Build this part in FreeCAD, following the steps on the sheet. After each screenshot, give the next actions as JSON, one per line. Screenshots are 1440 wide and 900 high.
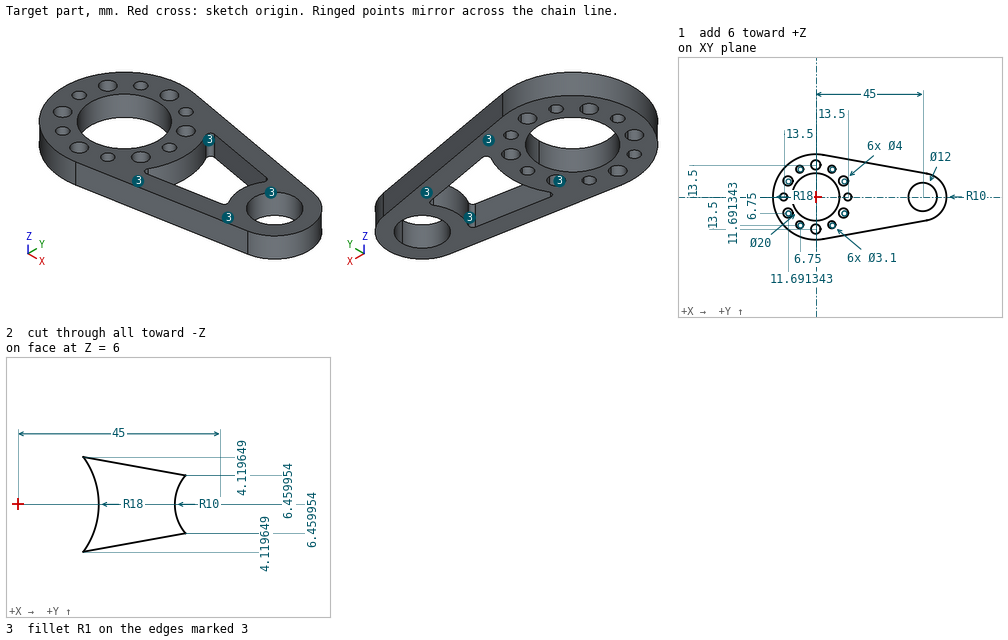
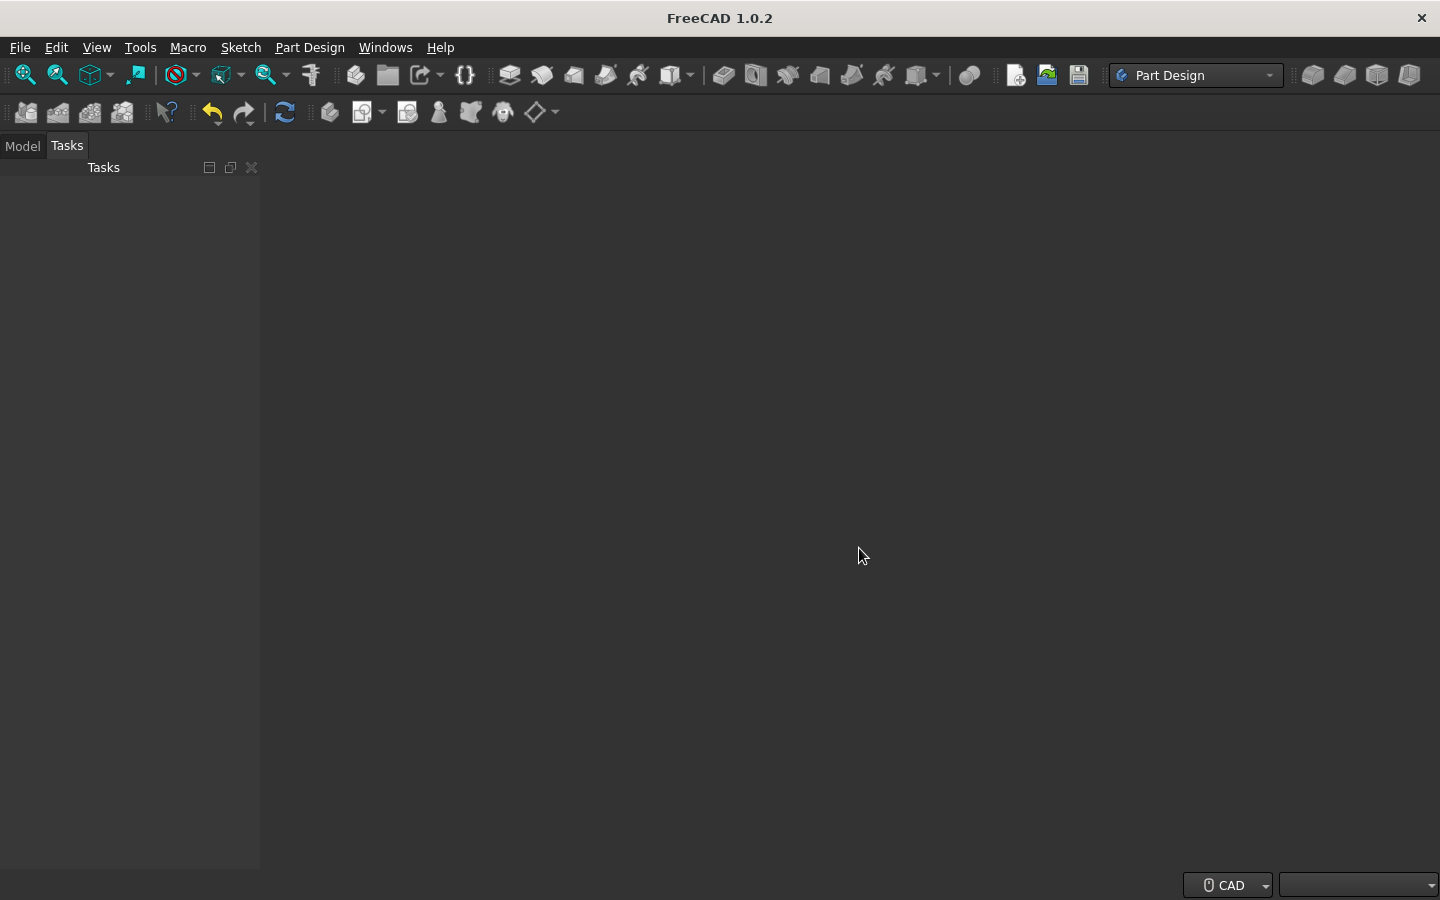
{"action": "left_click", "coordinate": [1016, 76]}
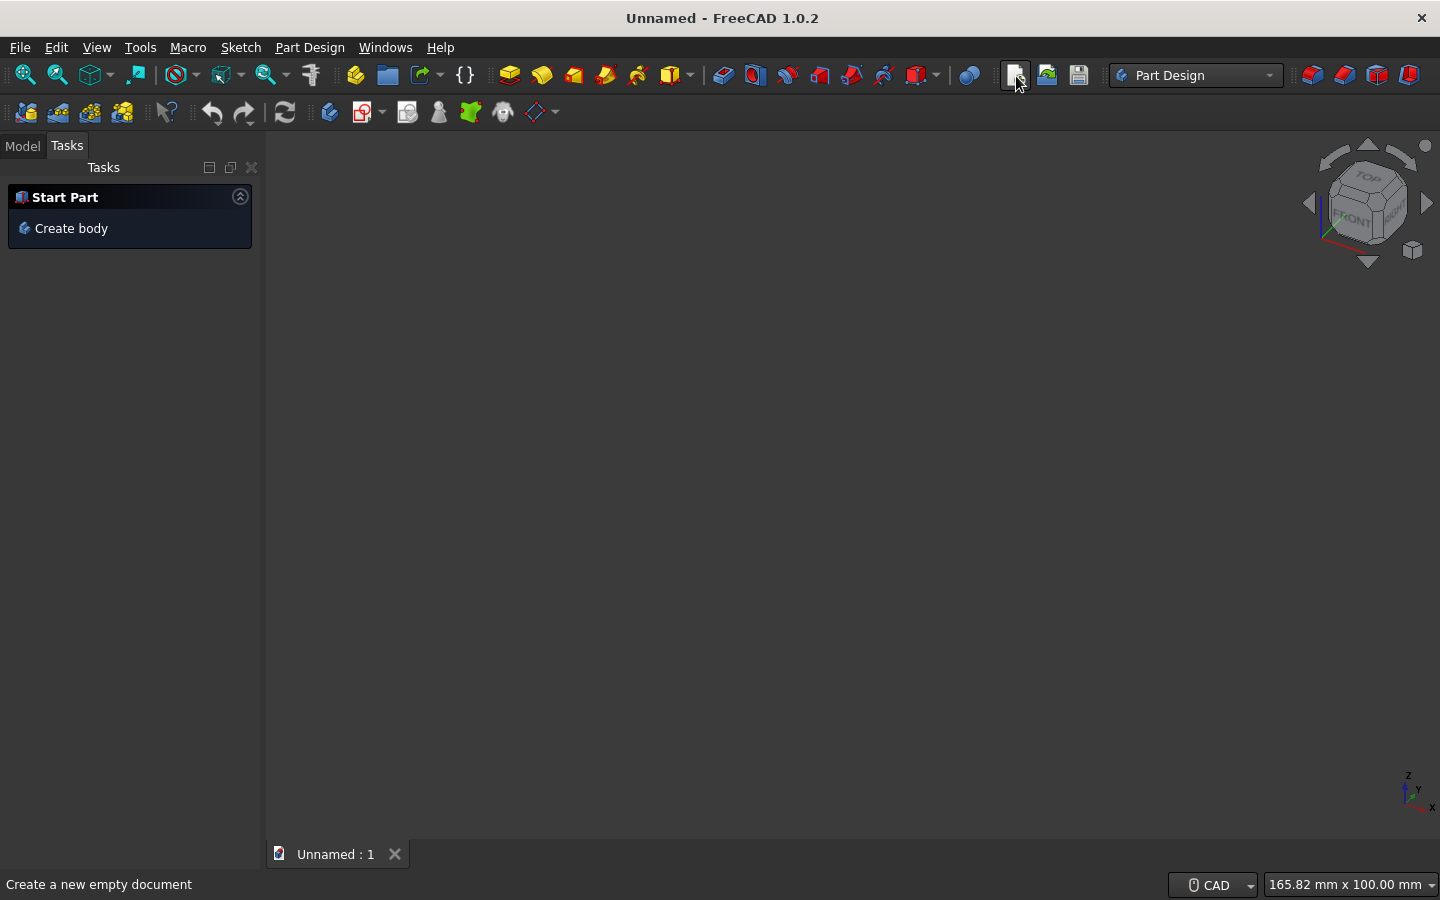
{"action": "left_click", "coordinate": [362, 112]}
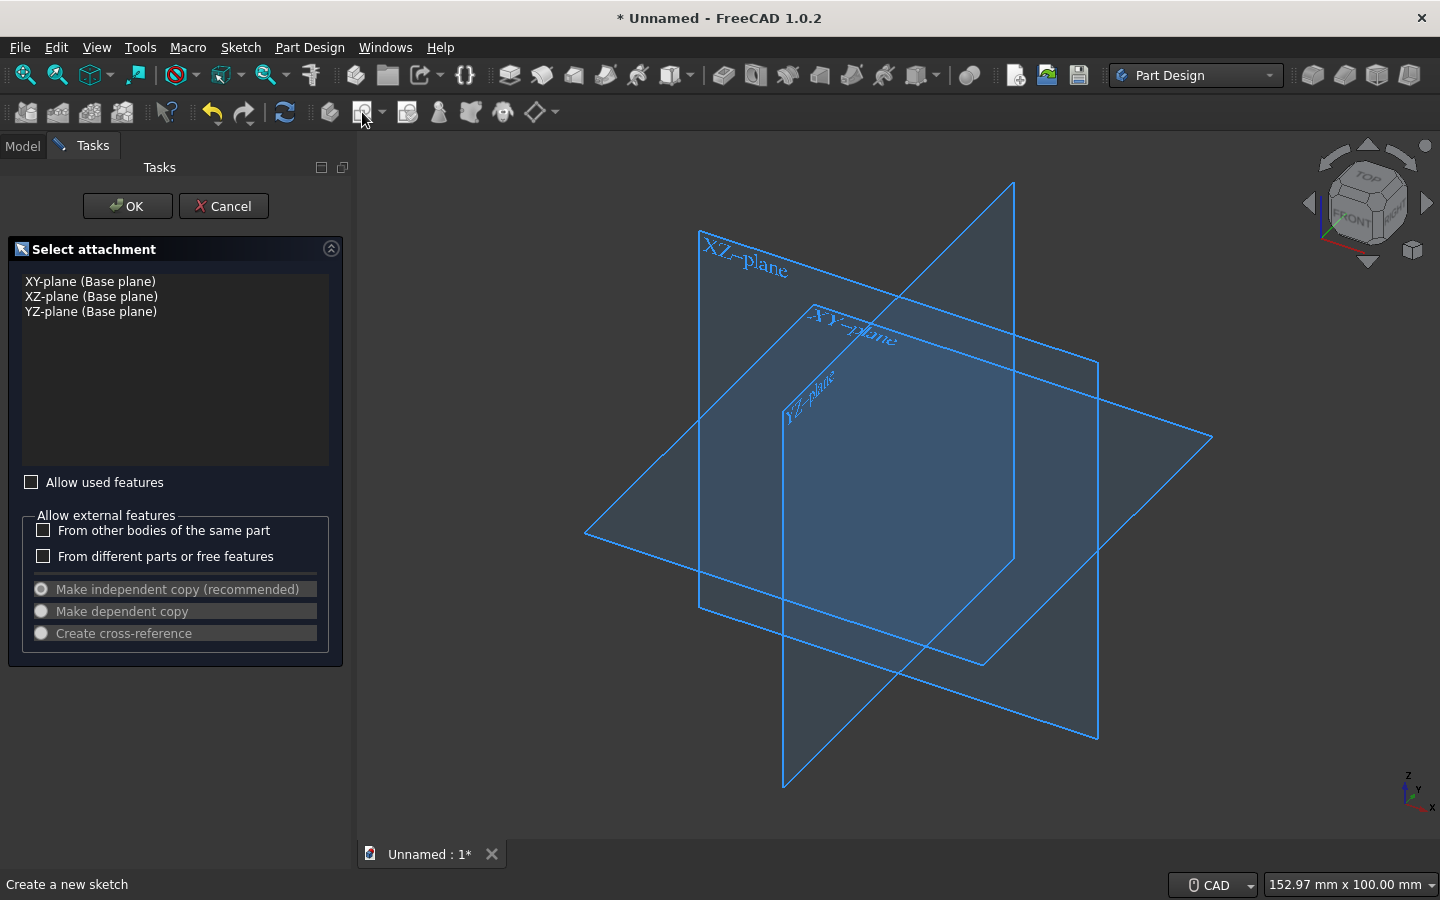
{"action": "left_click", "coordinate": [82, 282]}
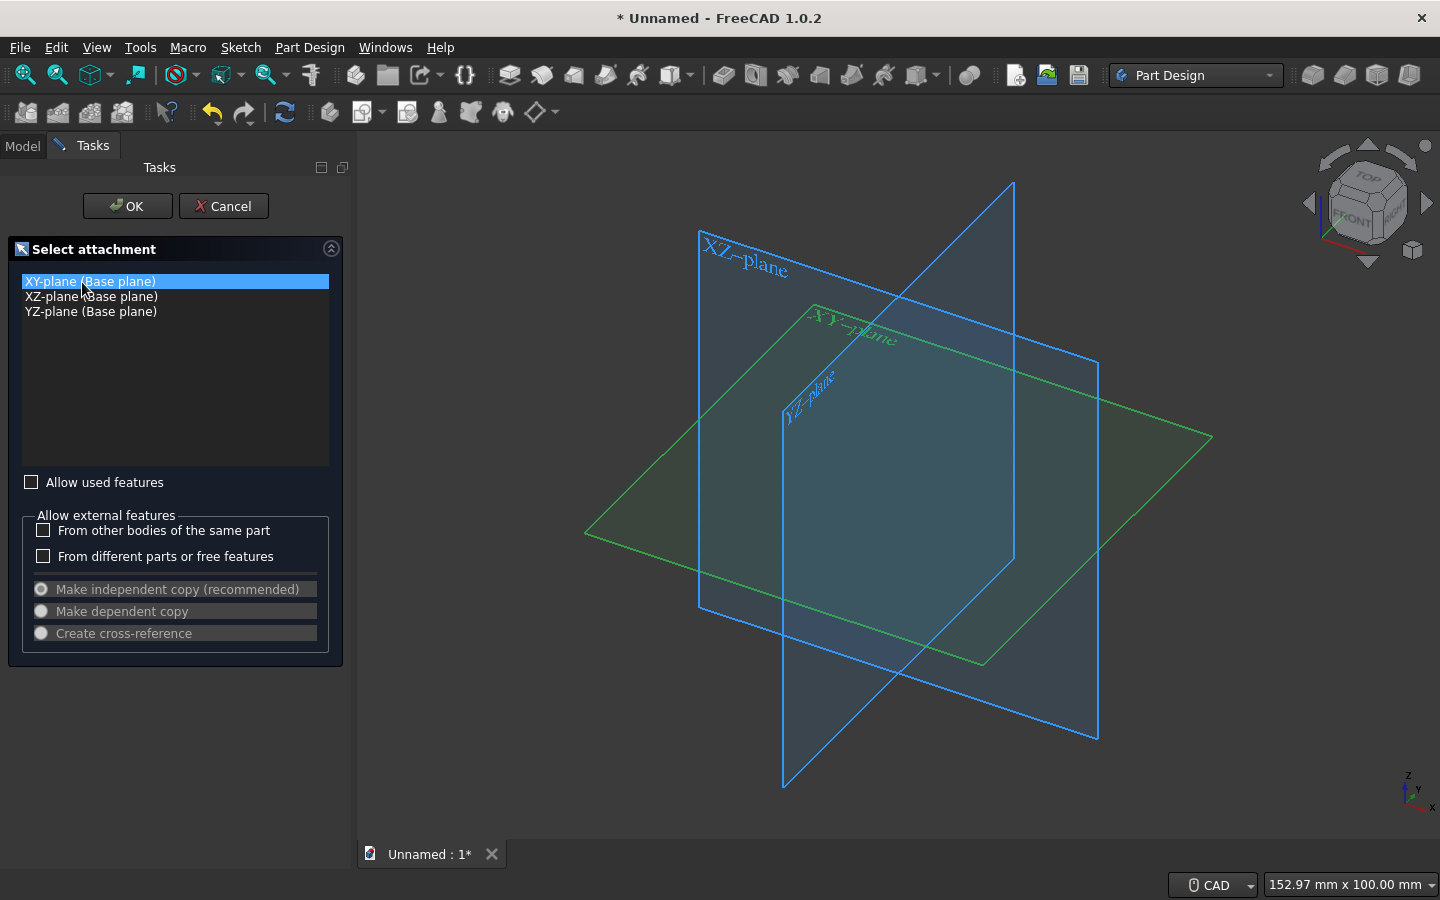
{"action": "left_click", "coordinate": [128, 206]}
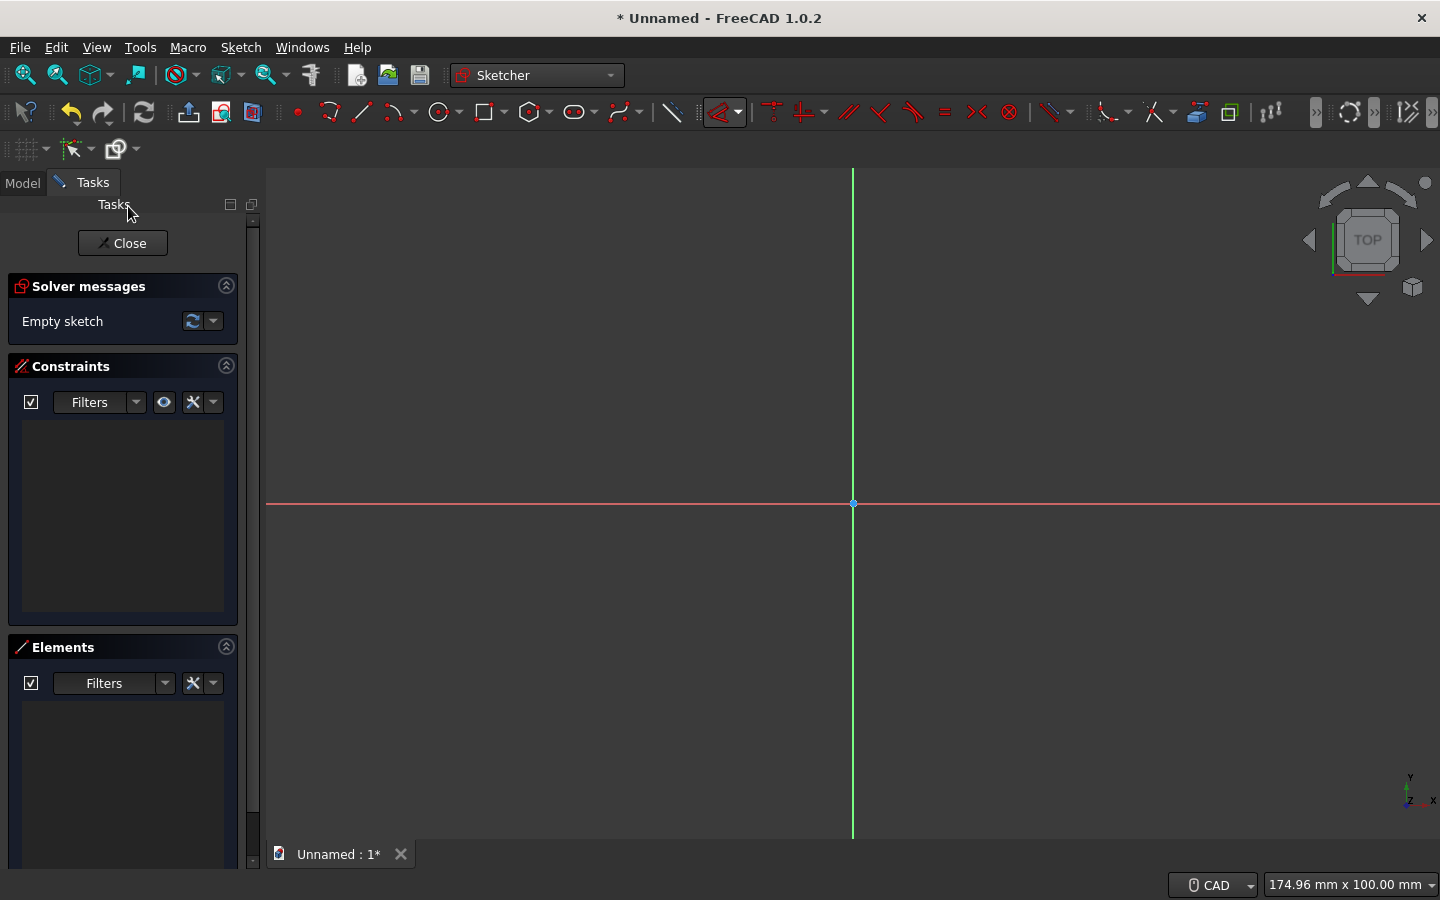
{"action": "scroll", "coordinate": [1275, 504], "scroll_direction": "up", "scroll_amount": 2}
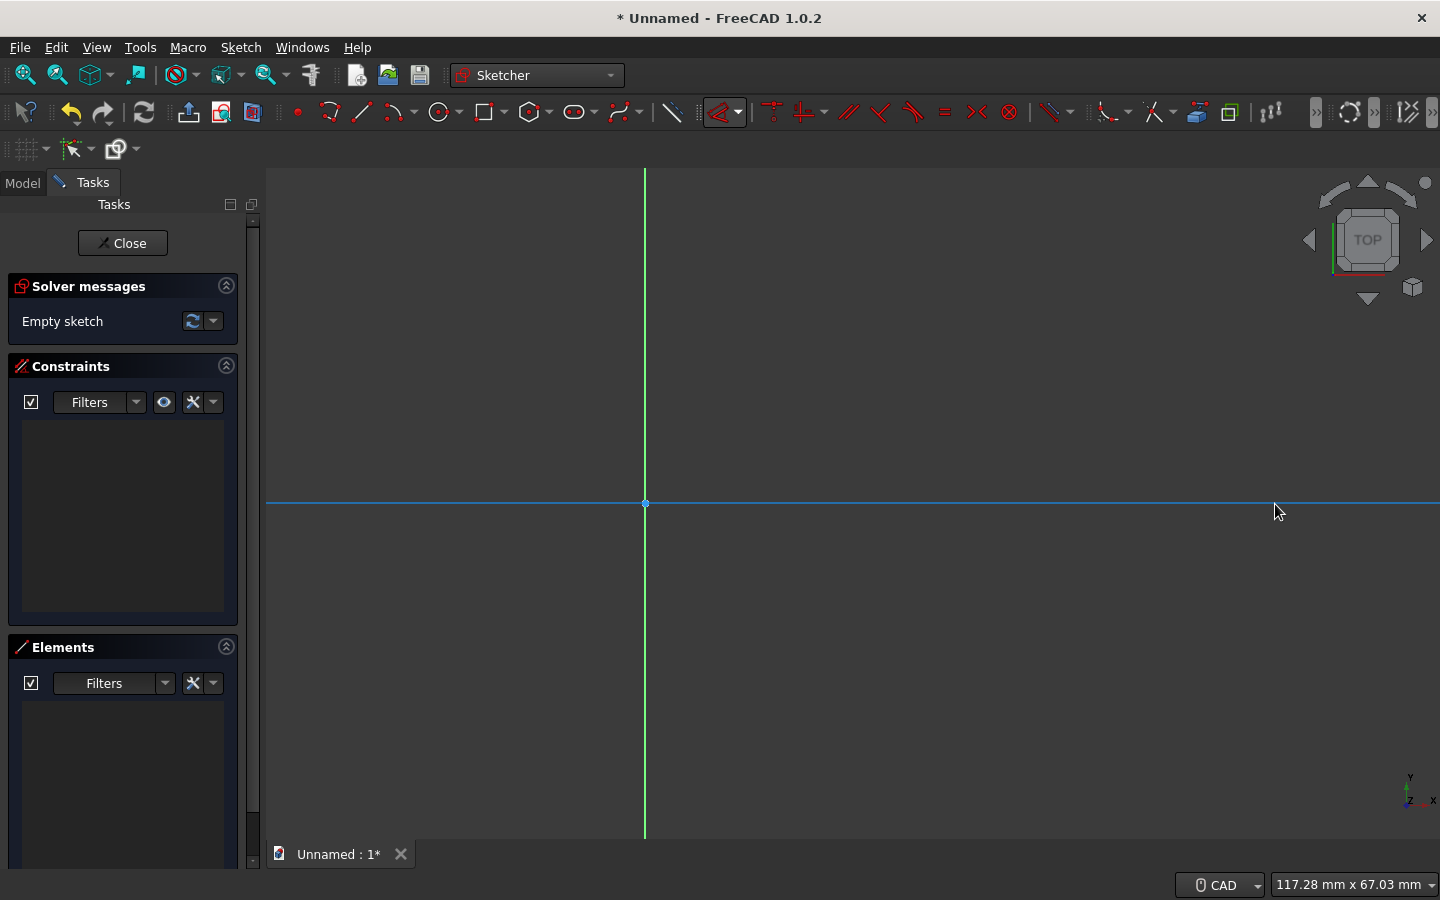
{"action": "left_click", "coordinate": [362, 112]}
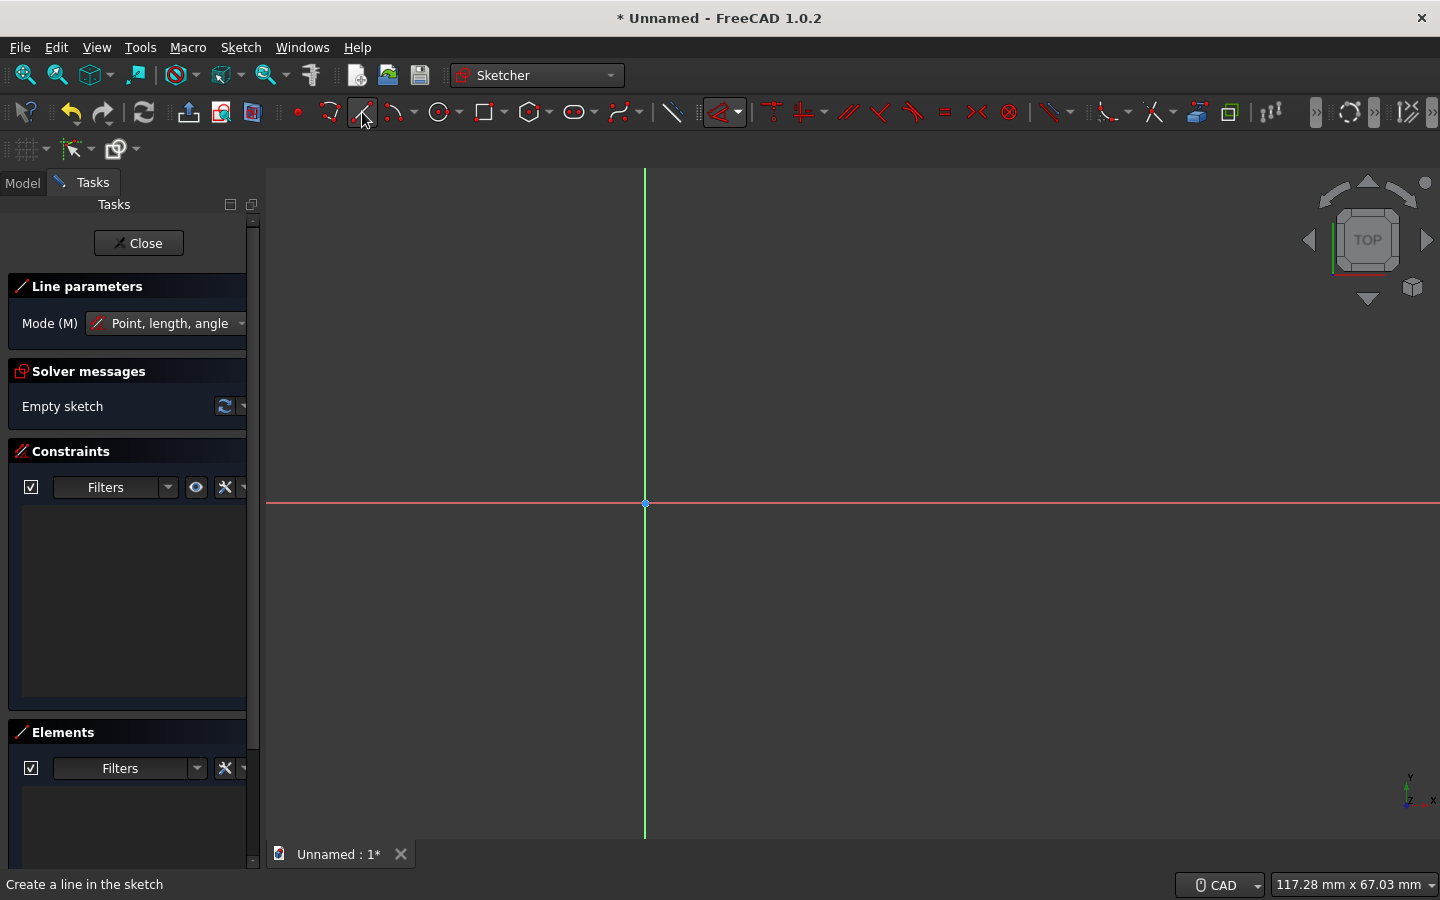
{"action": "left_click", "coordinate": [1113, 405]}
{"action": "left_click", "coordinate": [677, 326]}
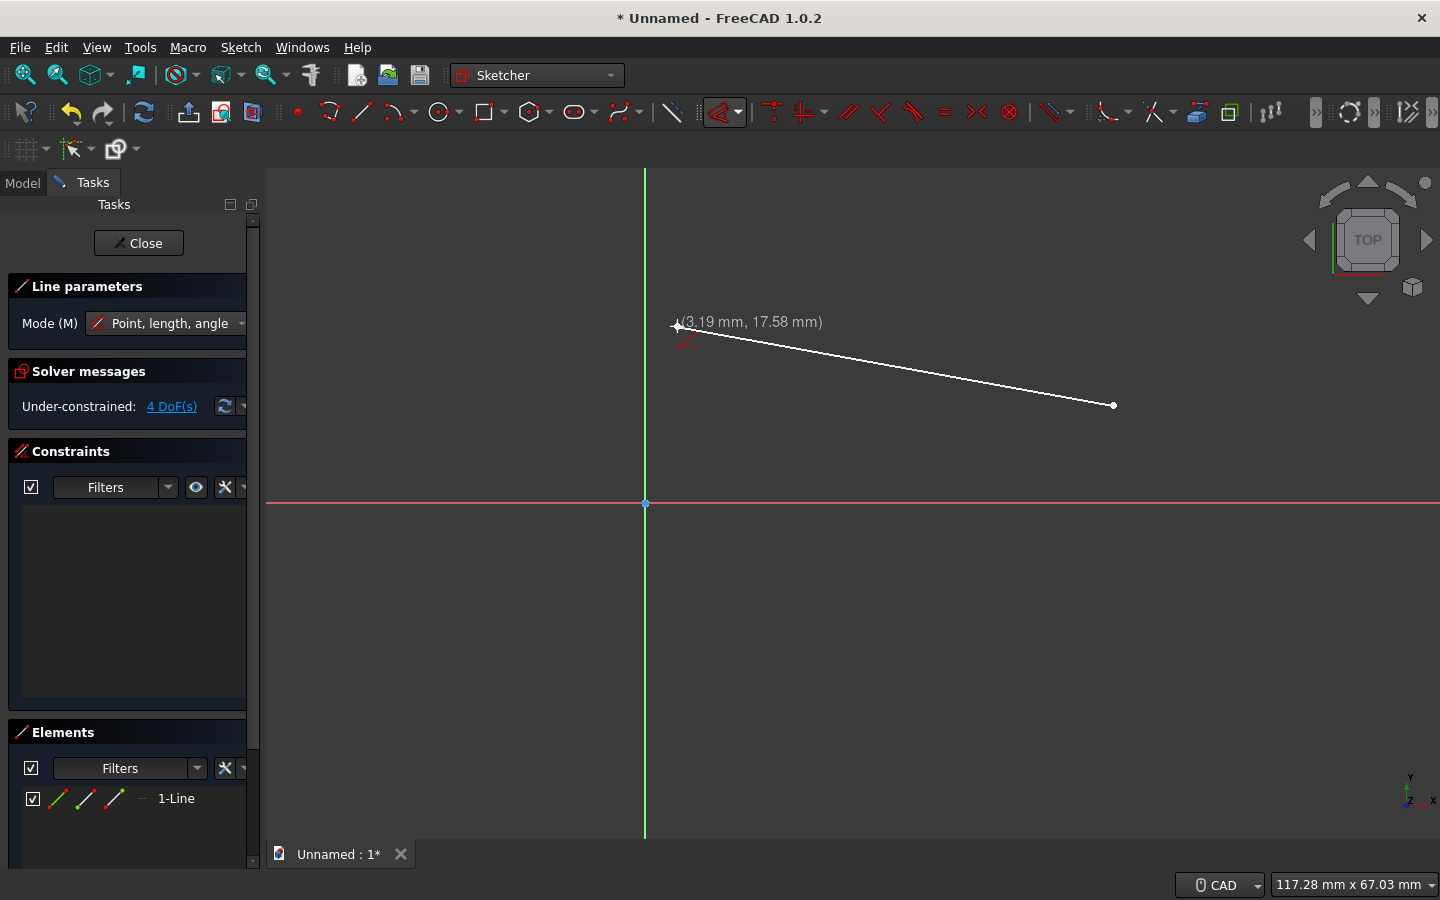
{"action": "left_click", "coordinate": [677, 680]}
{"action": "left_click", "coordinate": [1113, 602]}